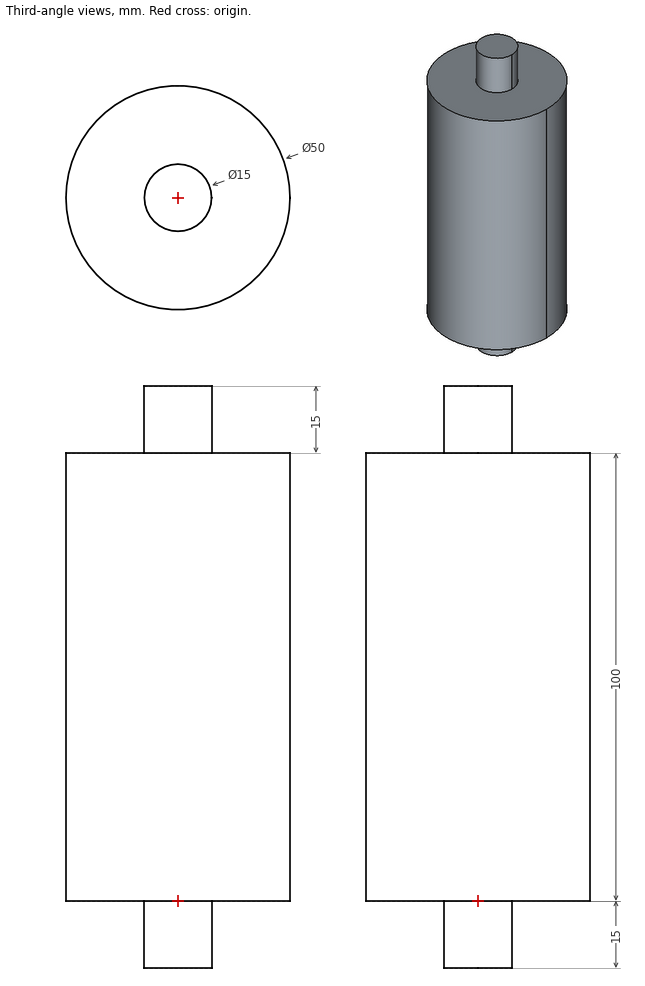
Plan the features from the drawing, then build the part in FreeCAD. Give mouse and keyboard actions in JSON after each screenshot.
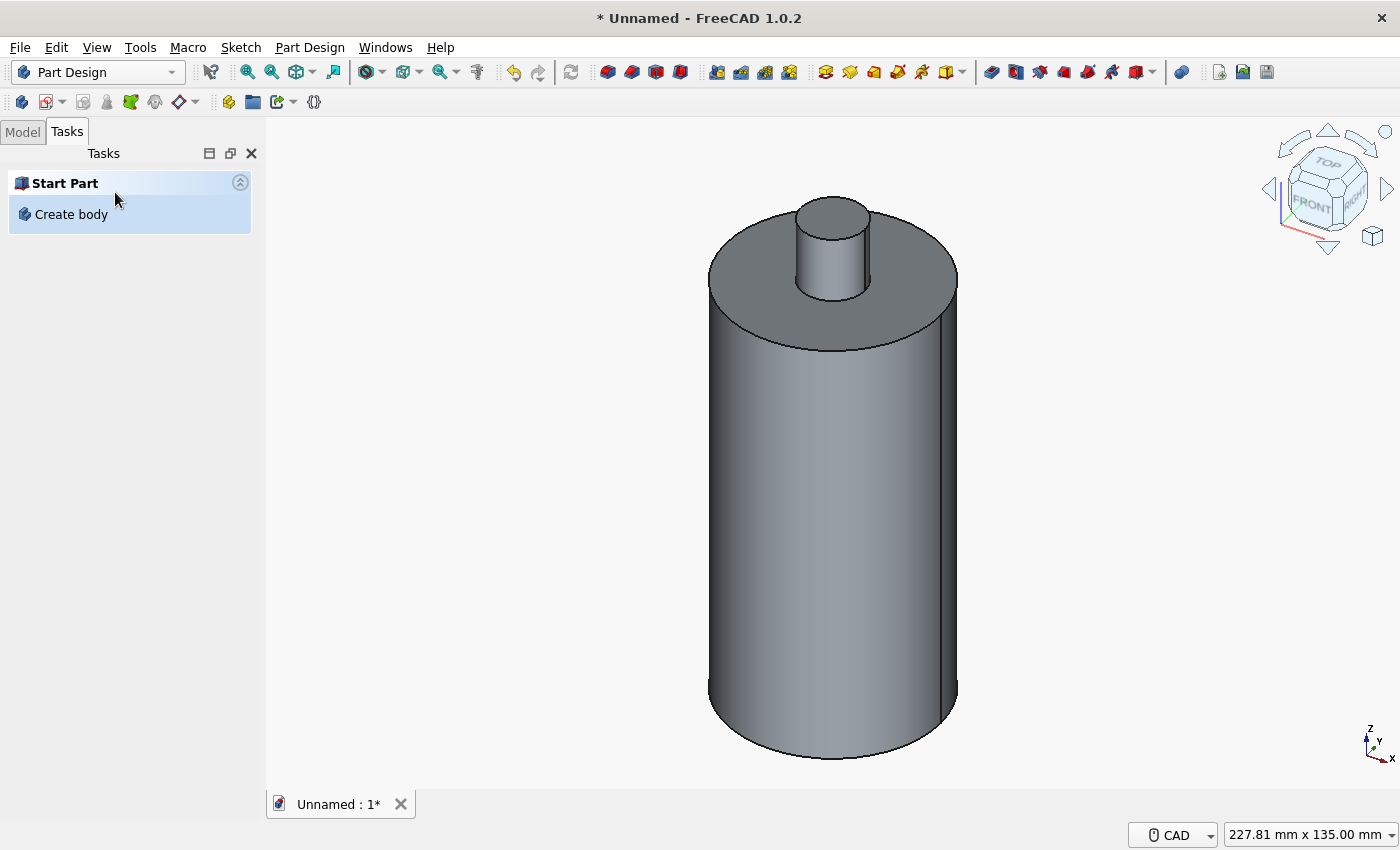
{"action": "left_click", "coordinate": [23, 131]}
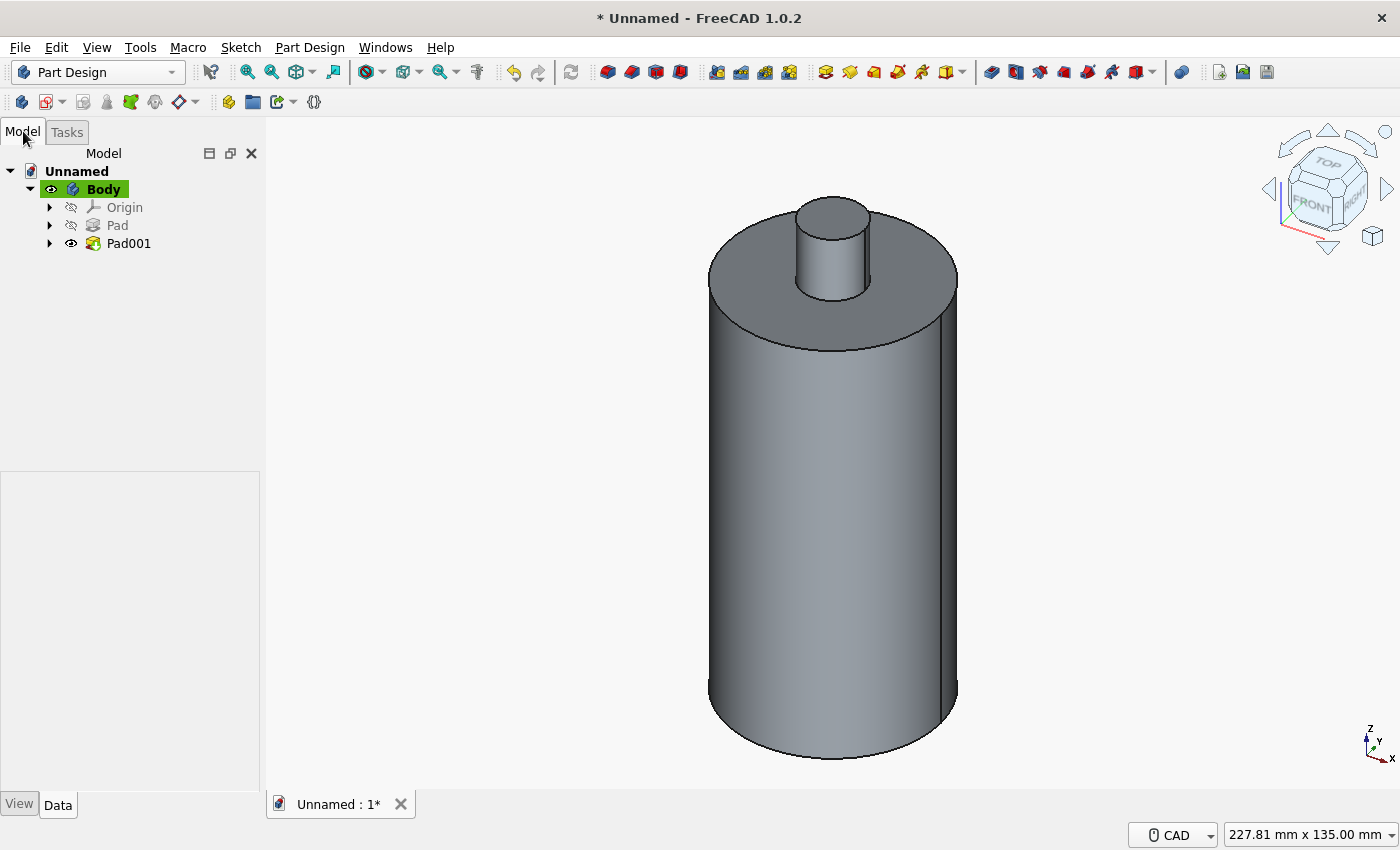
{"action": "left_click", "coordinate": [50, 207]}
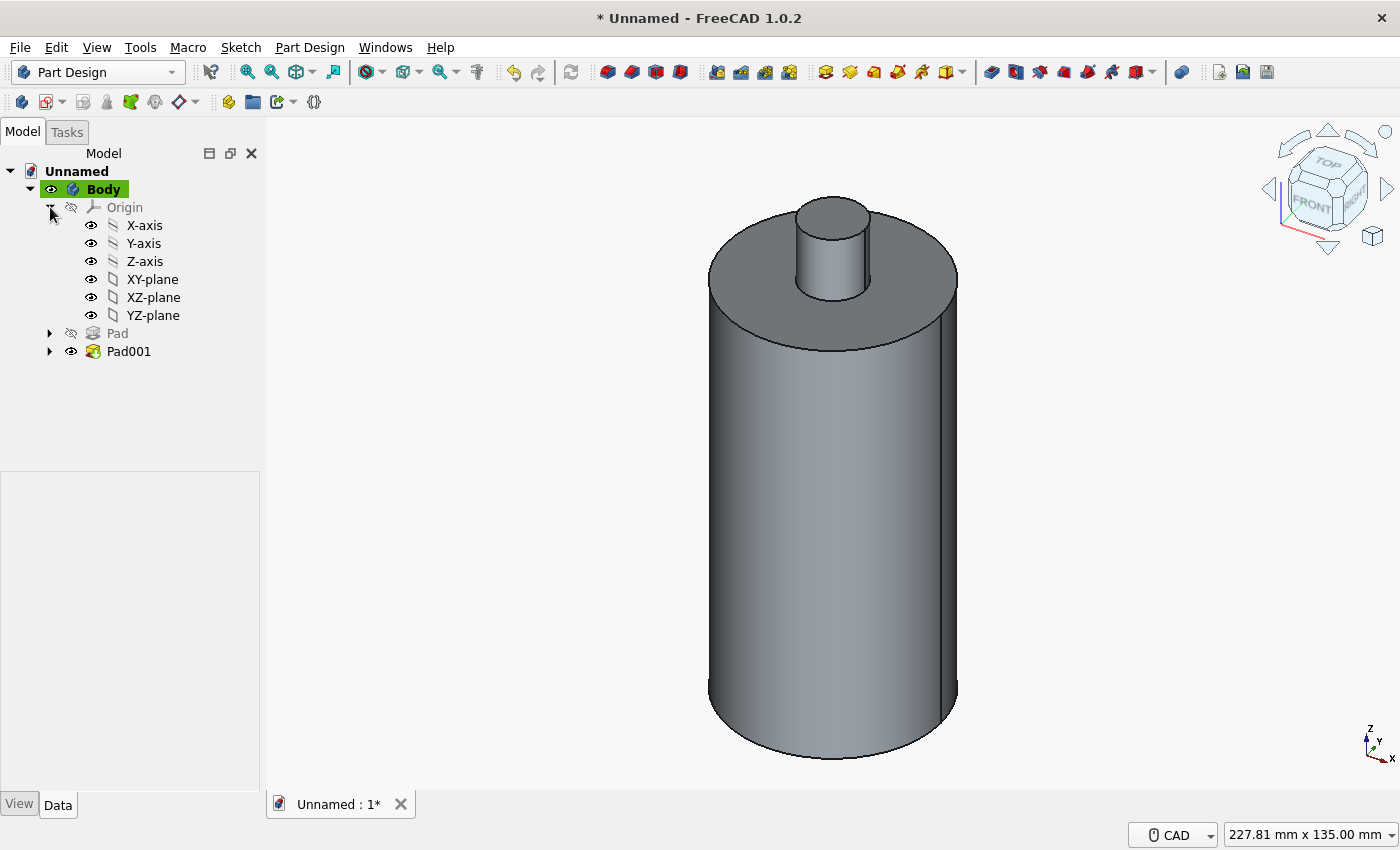
{"action": "left_click", "coordinate": [136, 279]}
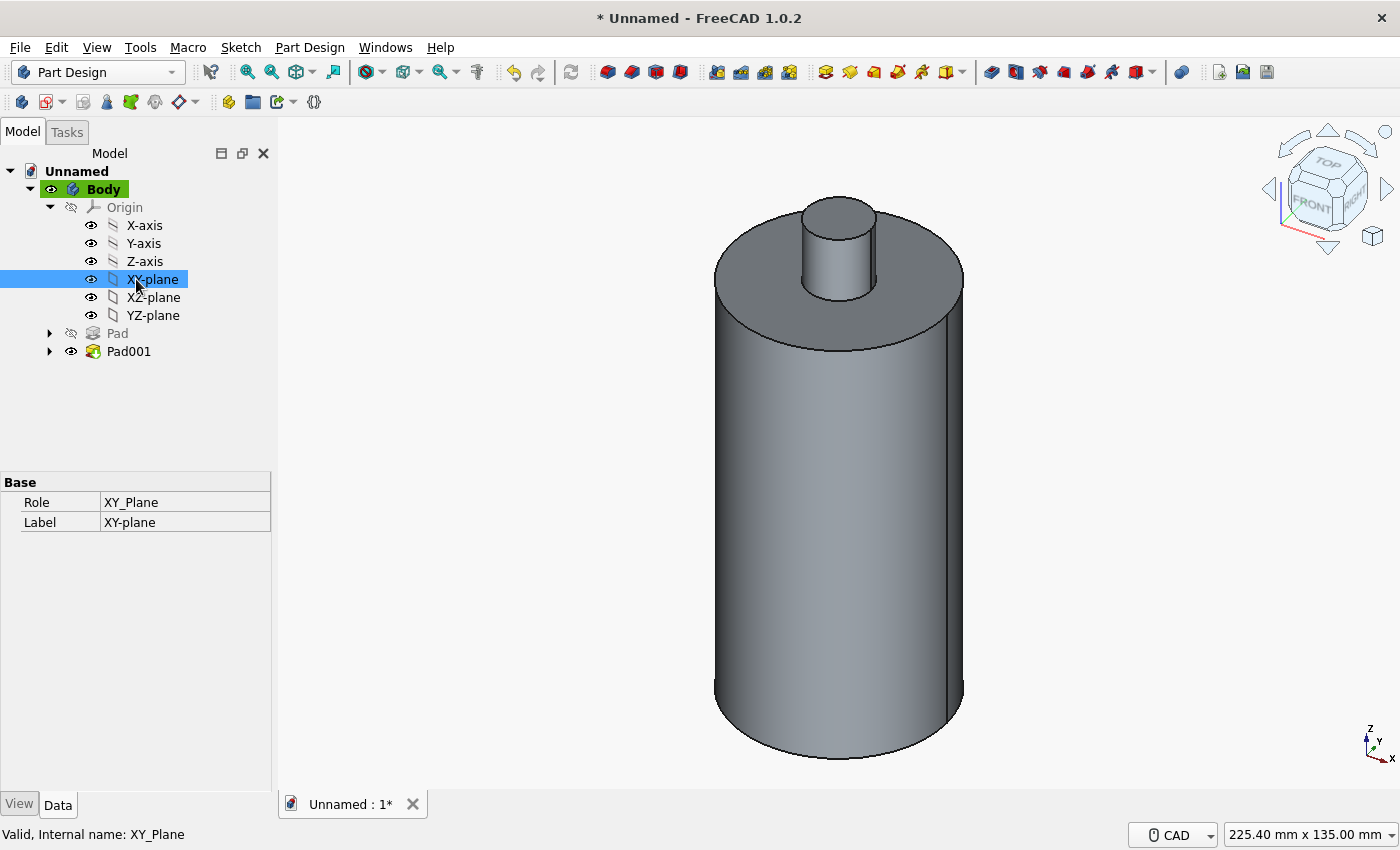
{"action": "left_click", "coordinate": [180, 102]}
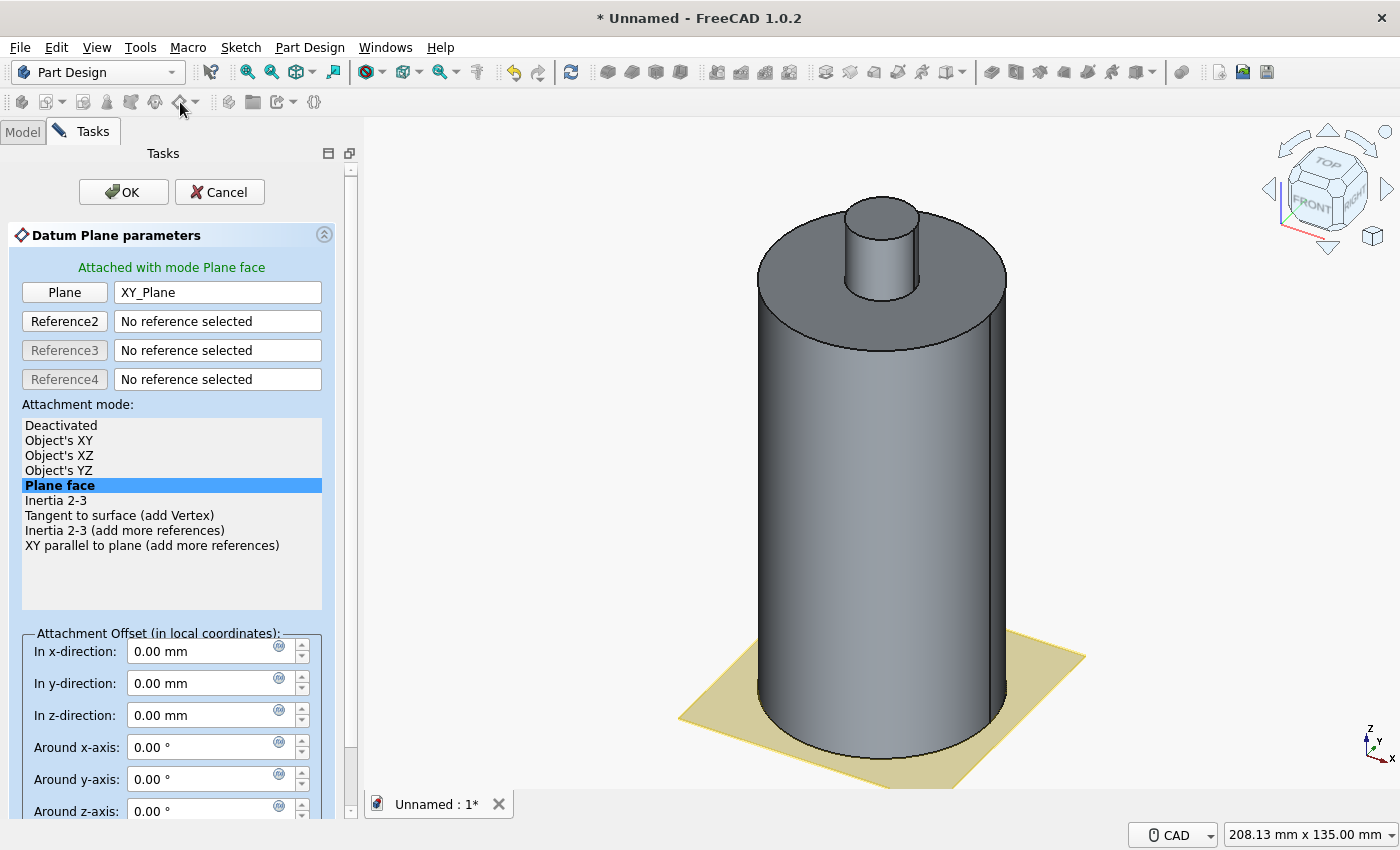
{"action": "triple_click", "coordinate": [210, 715]}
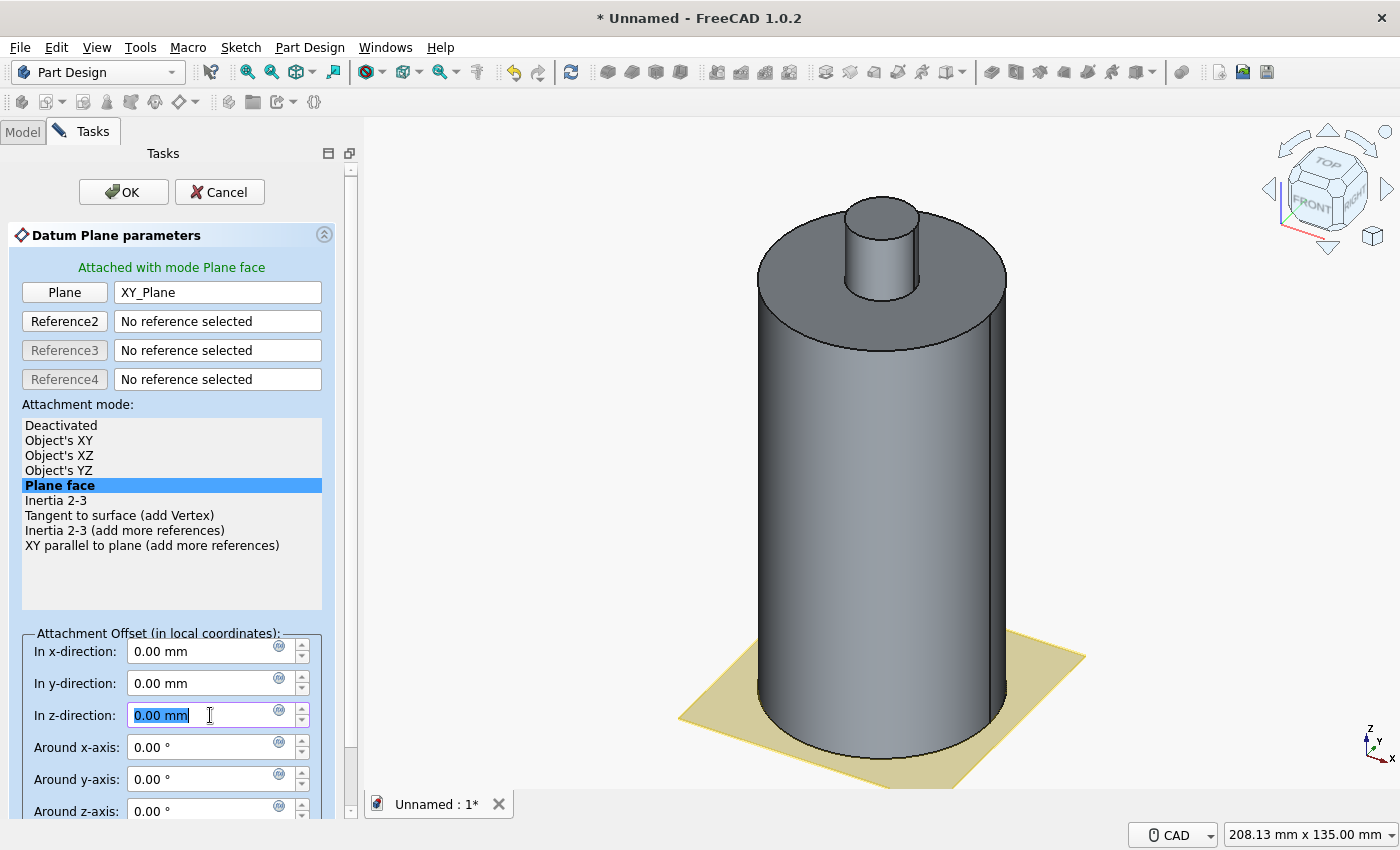
{"action": "type", "text": "-15"}
{"action": "key", "text": "Tab"}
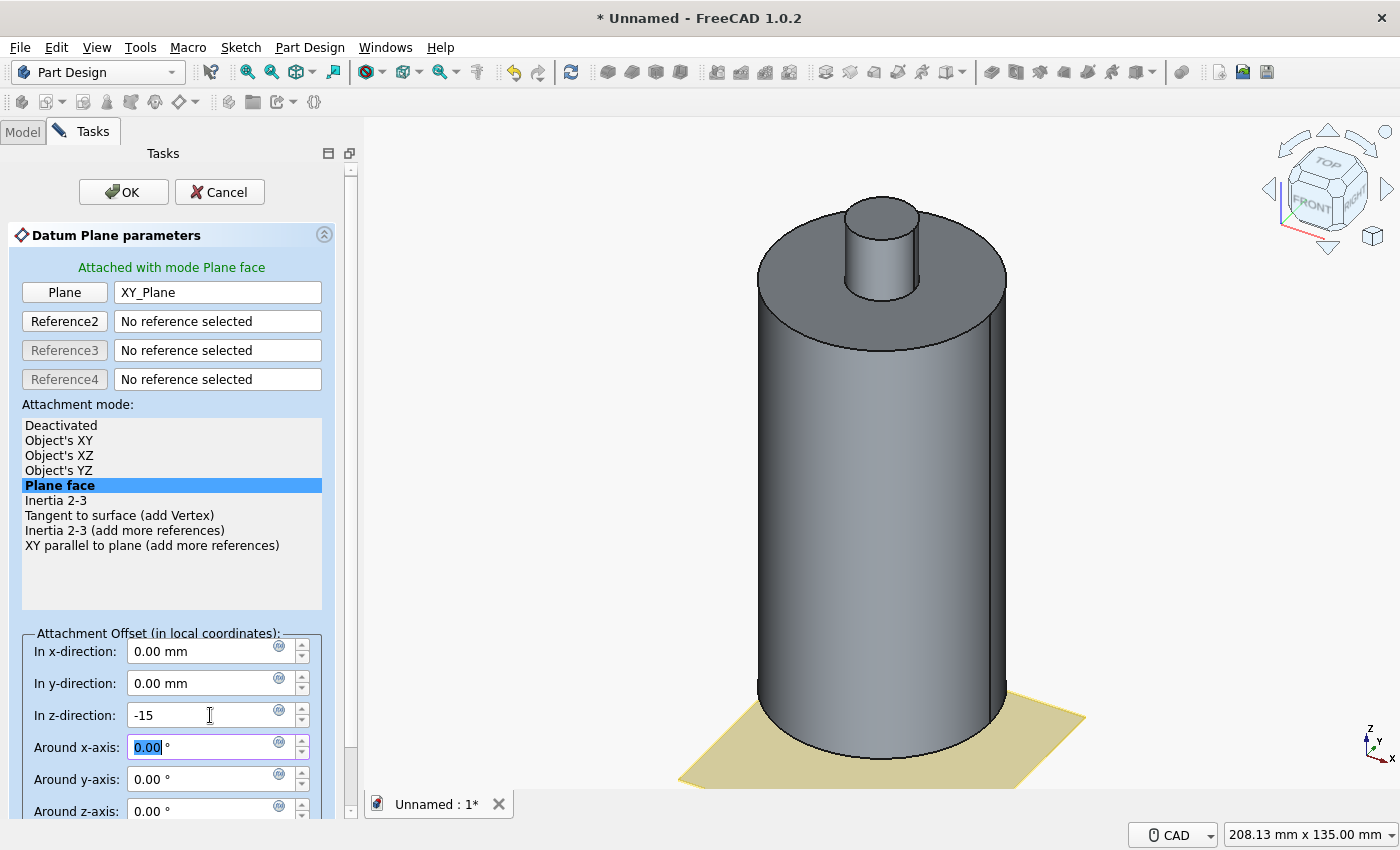
{"action": "left_click", "coordinate": [124, 192]}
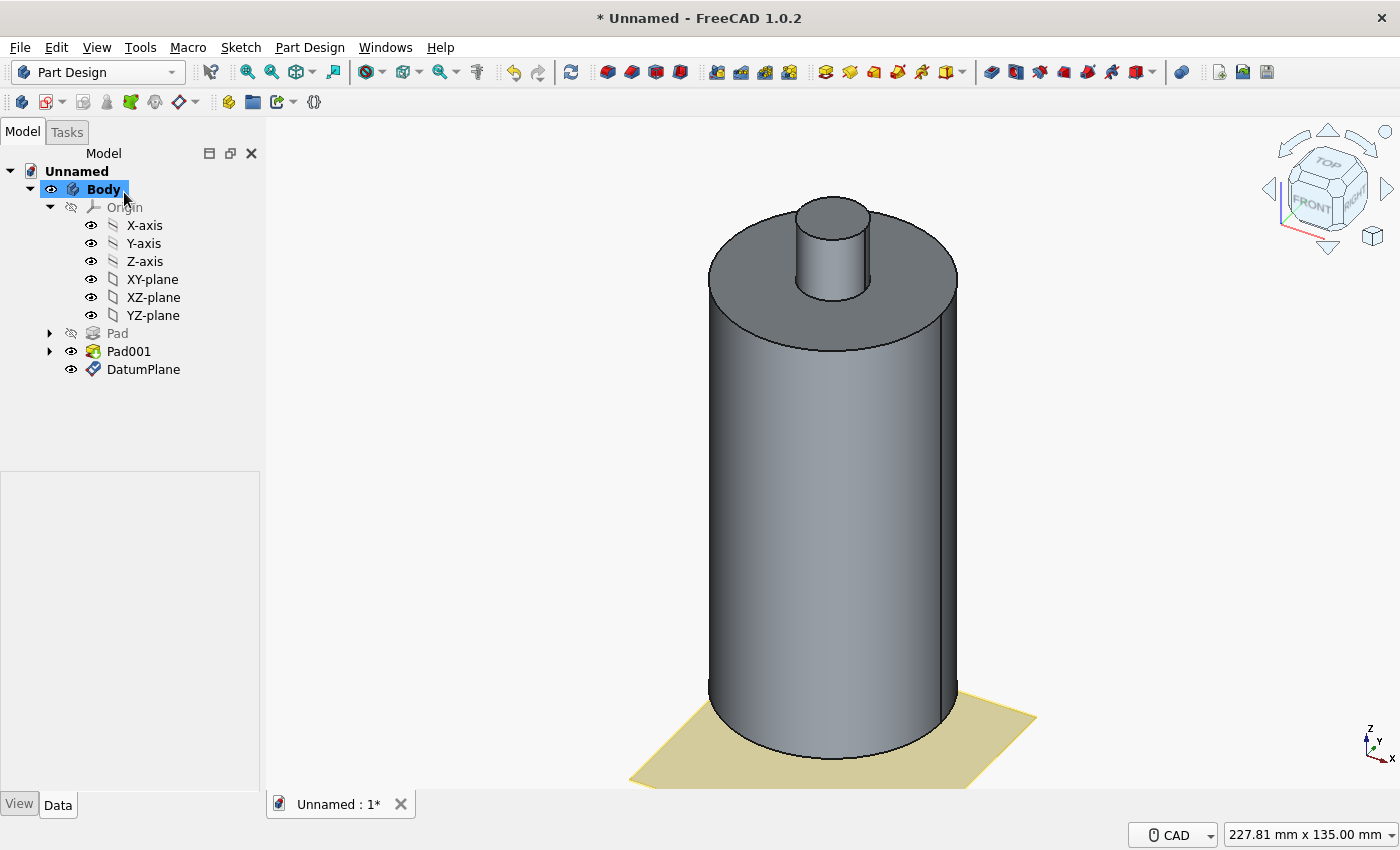
{"action": "left_click", "coordinate": [116, 369]}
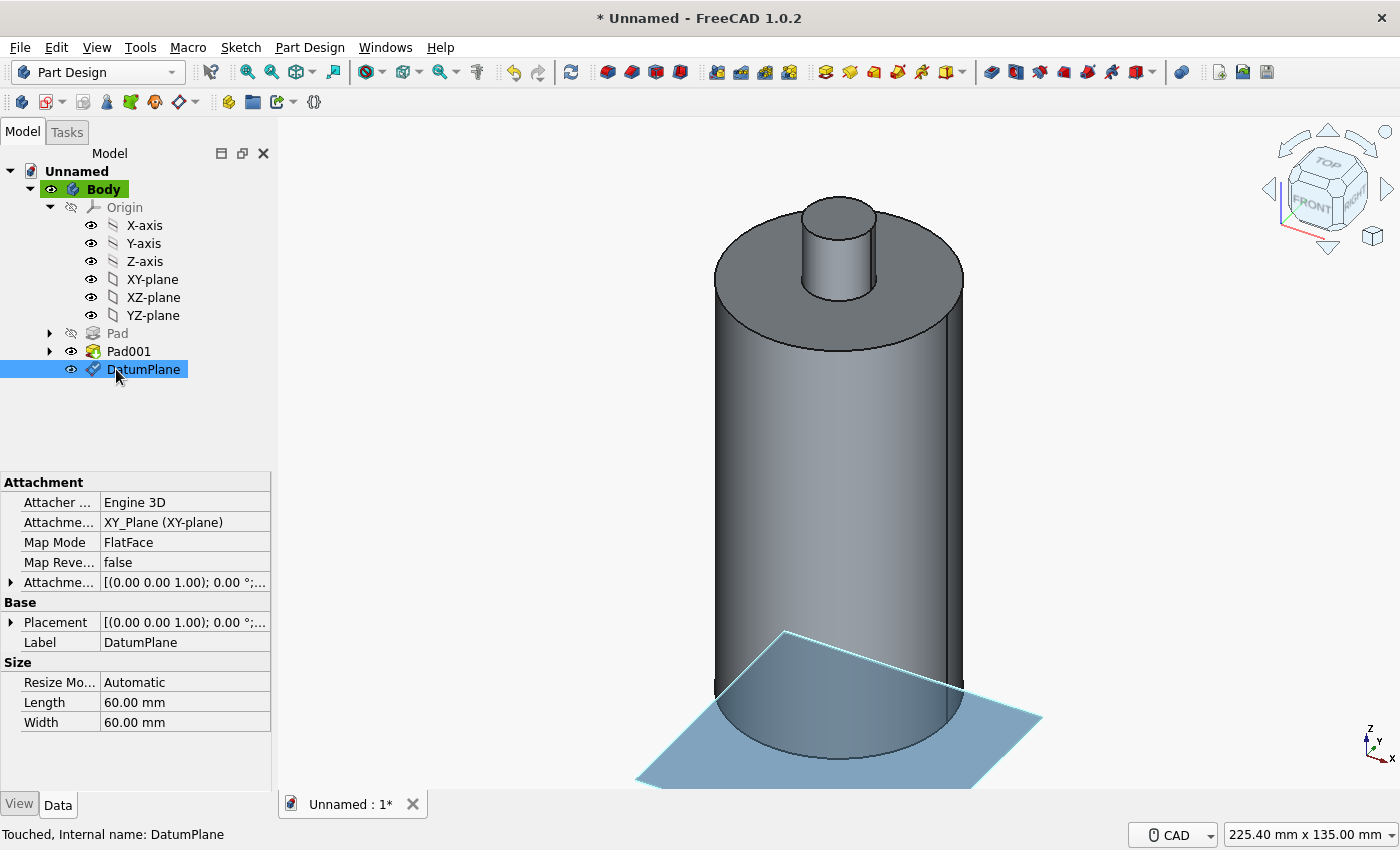
{"action": "left_click", "coordinate": [46, 102]}